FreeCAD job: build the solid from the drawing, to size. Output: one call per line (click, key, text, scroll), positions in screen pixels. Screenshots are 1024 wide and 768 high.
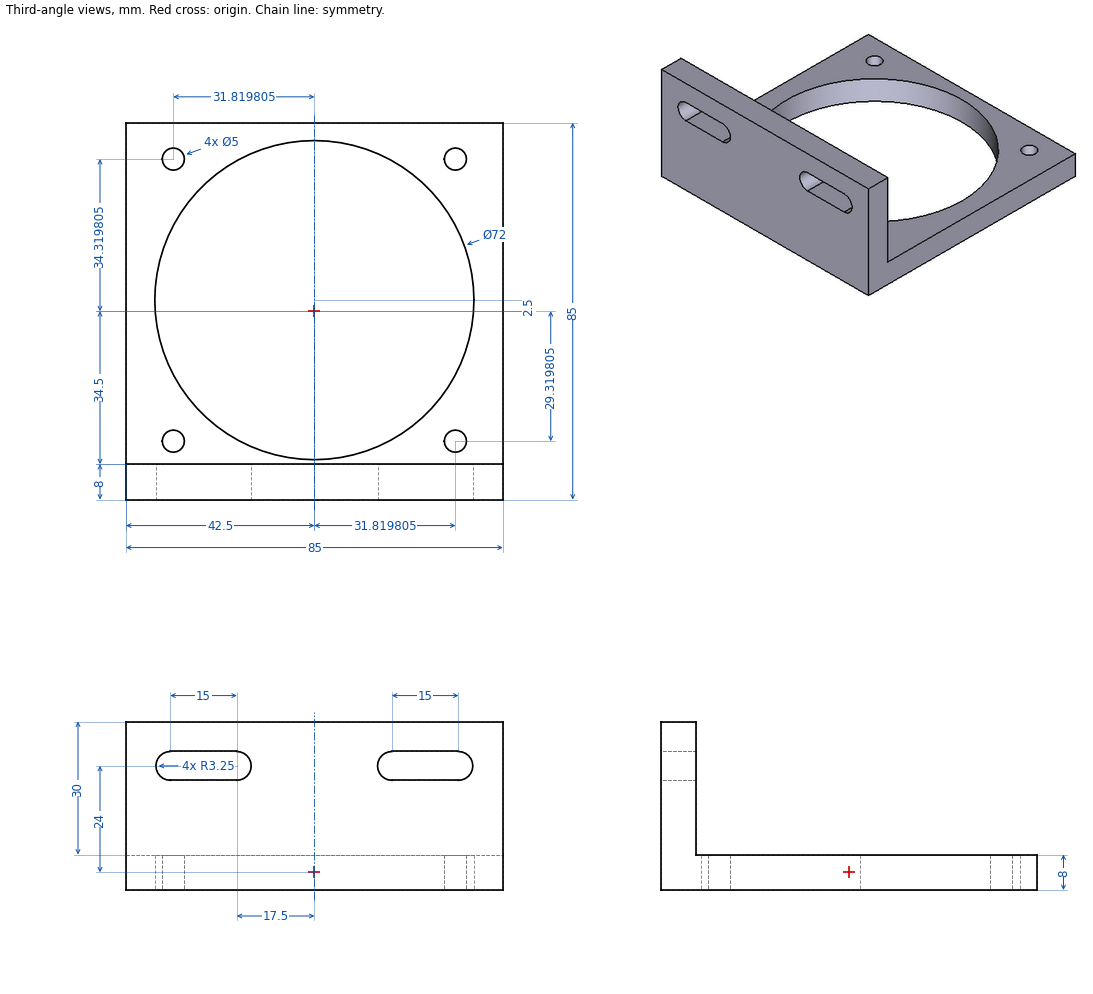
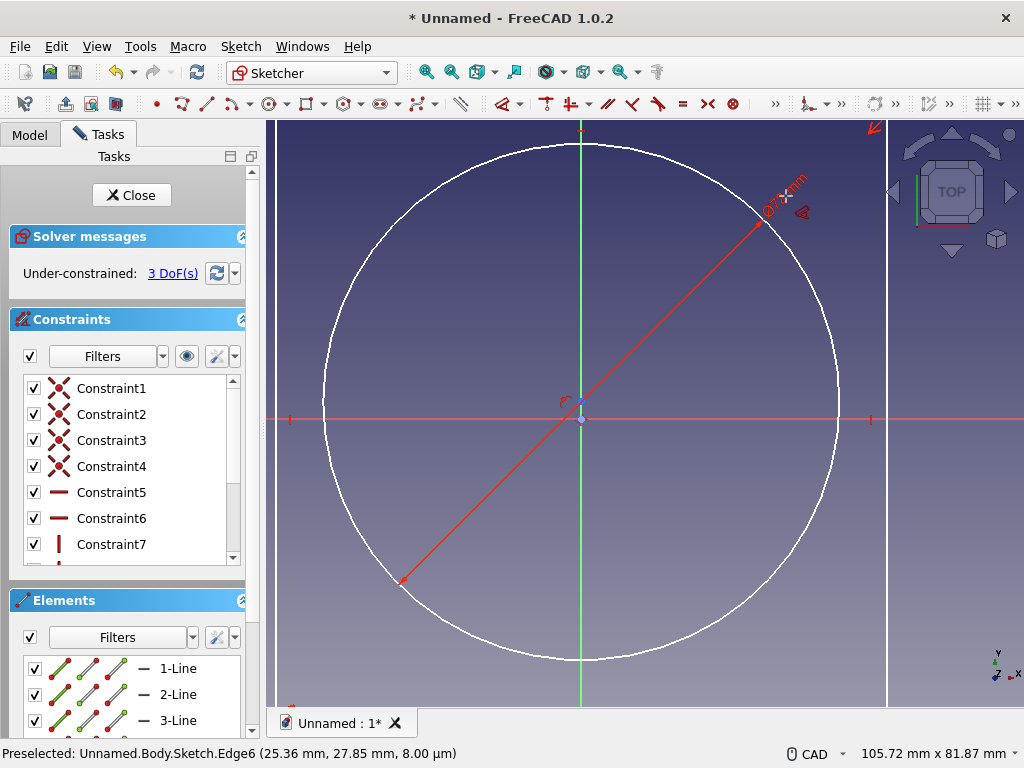
scroll(567, 401, down, 2)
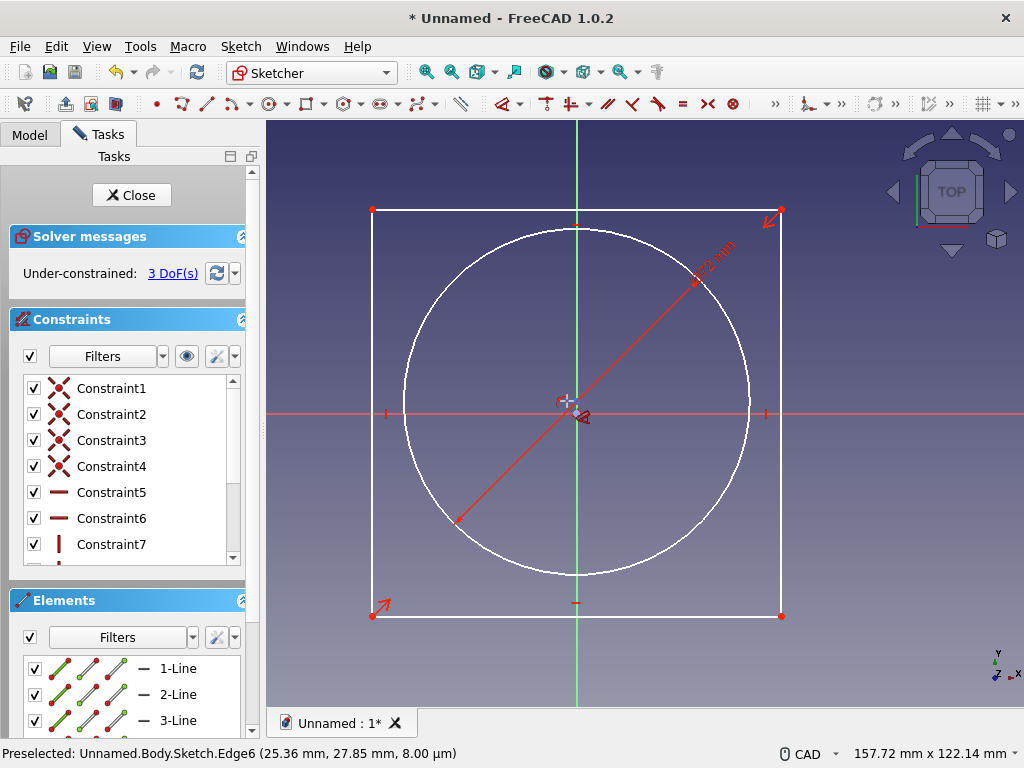
click(495, 617)
click(483, 651)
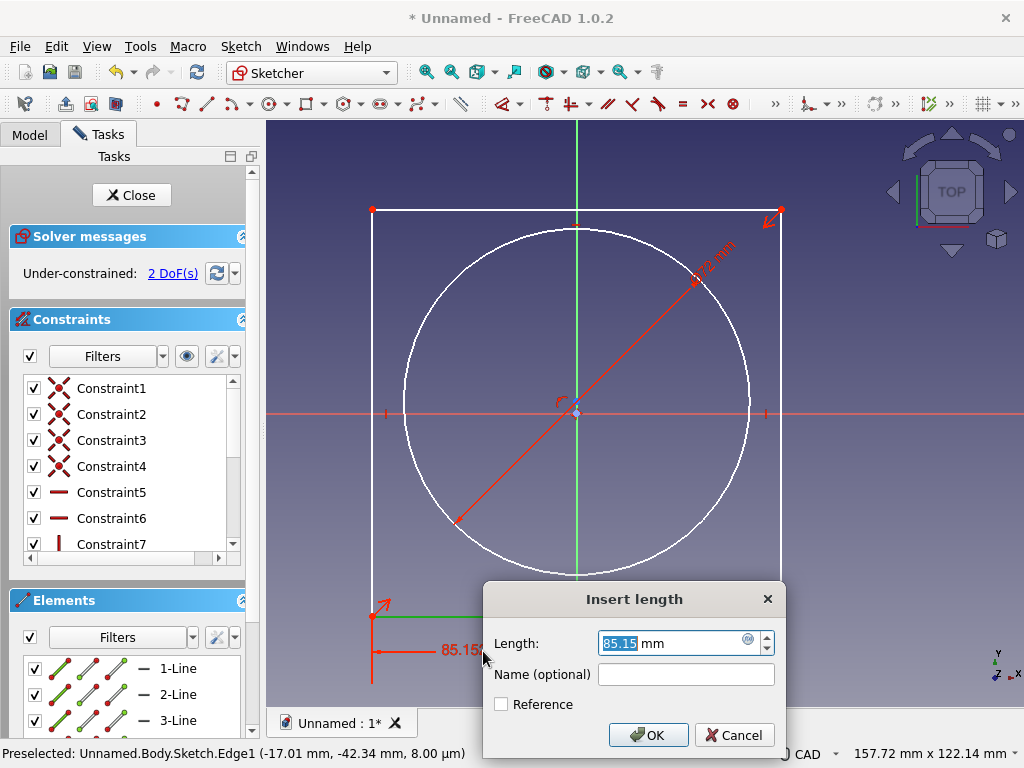
text(85)
key(Return)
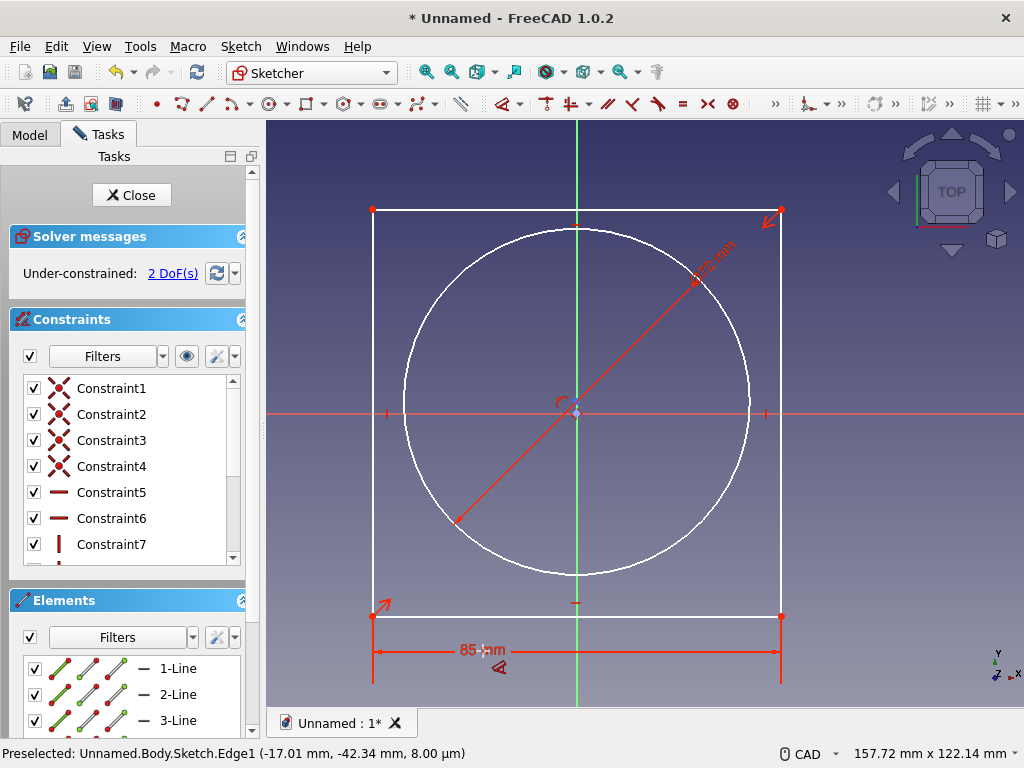
click(781, 495)
click(815, 320)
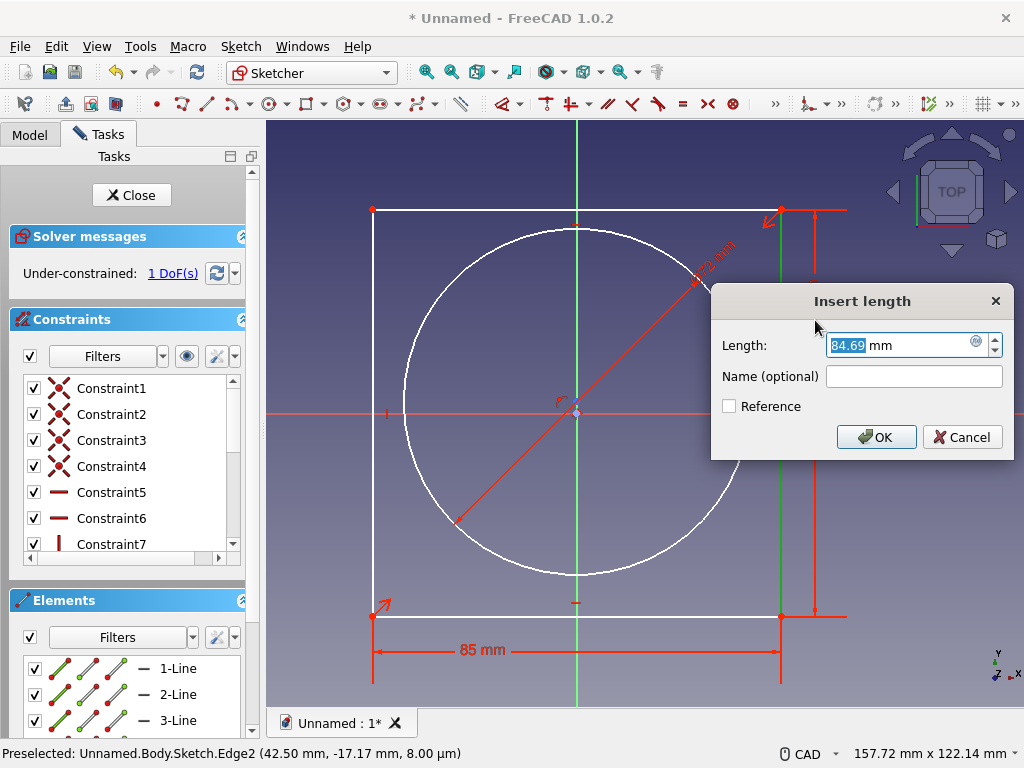
text(85)
key(Return)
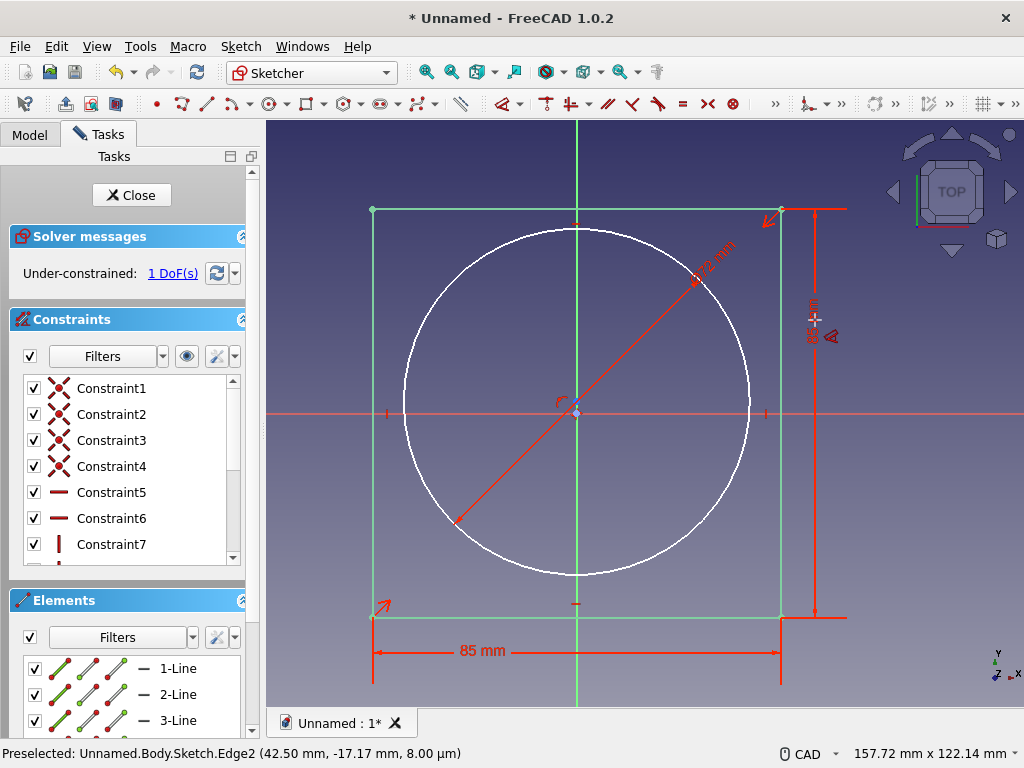
scroll(577, 402, up, 6)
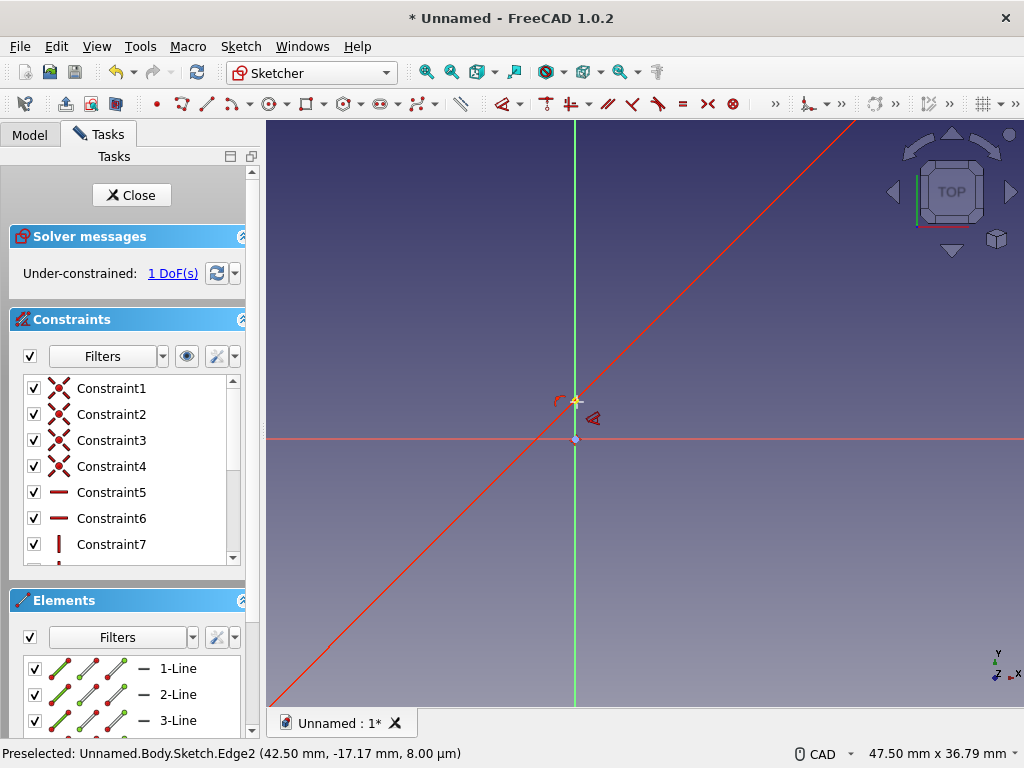
click(575, 400)
click(609, 420)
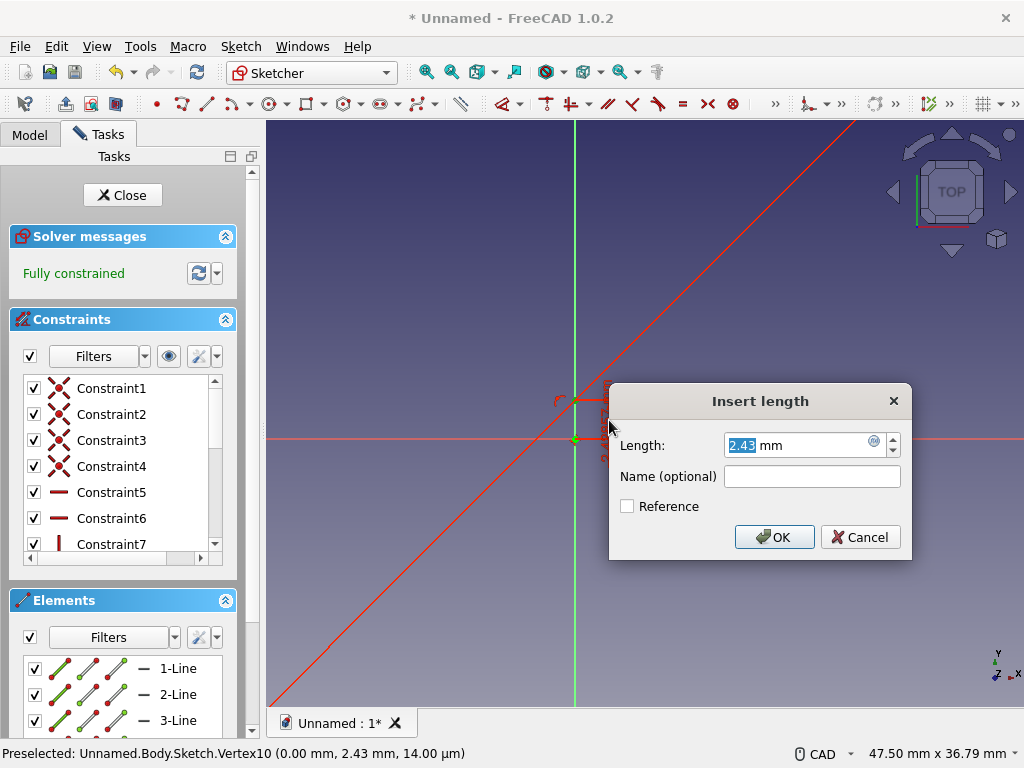
text(2.5)
key(Return)
key(Escape)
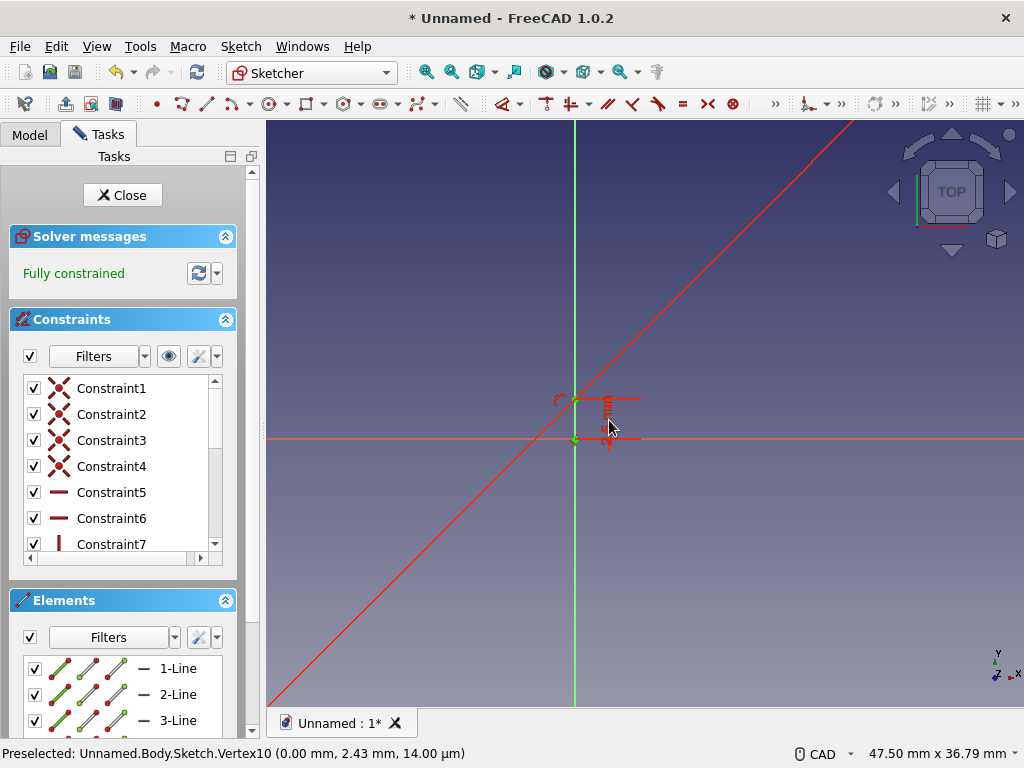
click(123, 195)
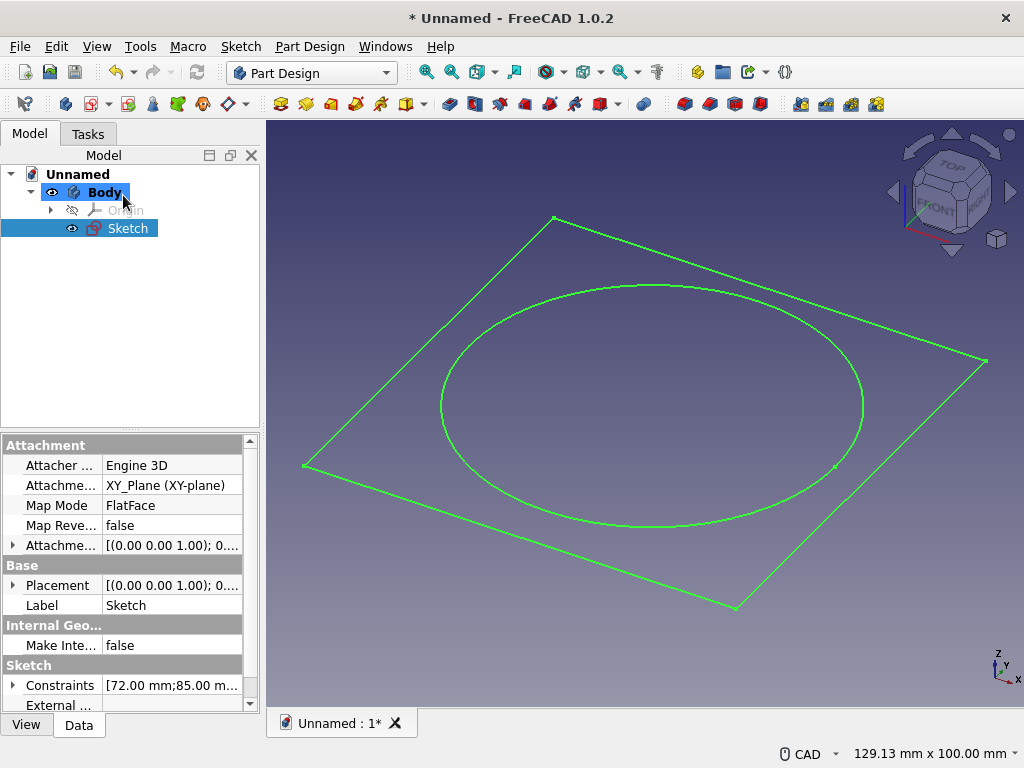
click(281, 104)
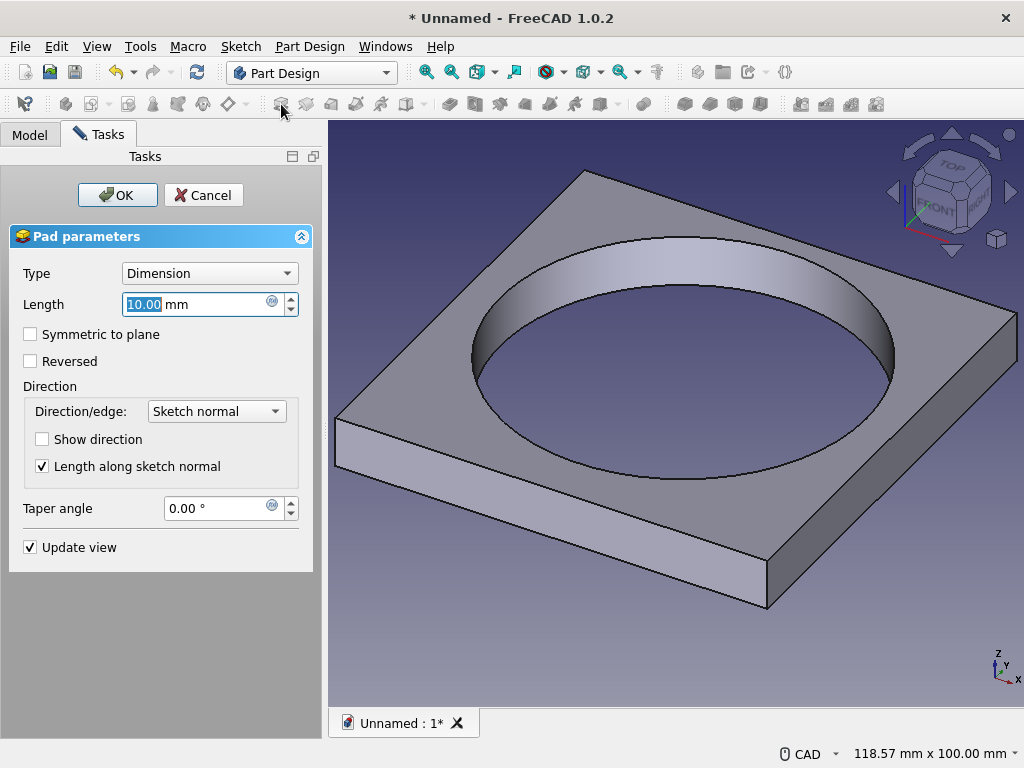
text(8)
key(Tab)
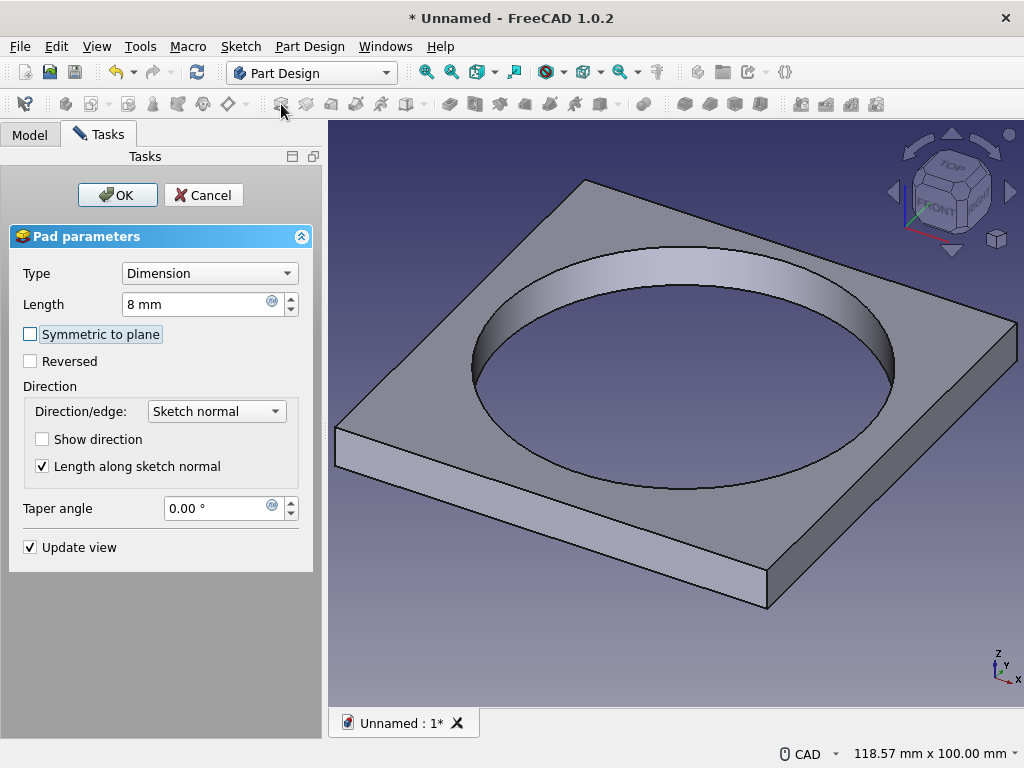
click(31, 334)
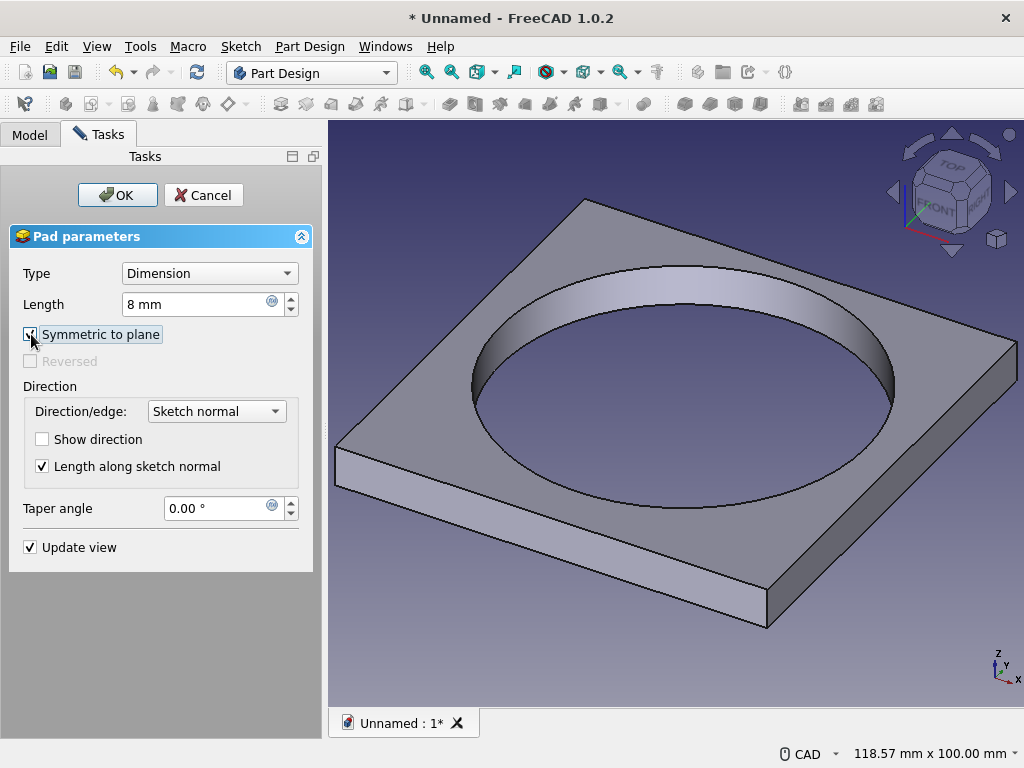
click(118, 195)